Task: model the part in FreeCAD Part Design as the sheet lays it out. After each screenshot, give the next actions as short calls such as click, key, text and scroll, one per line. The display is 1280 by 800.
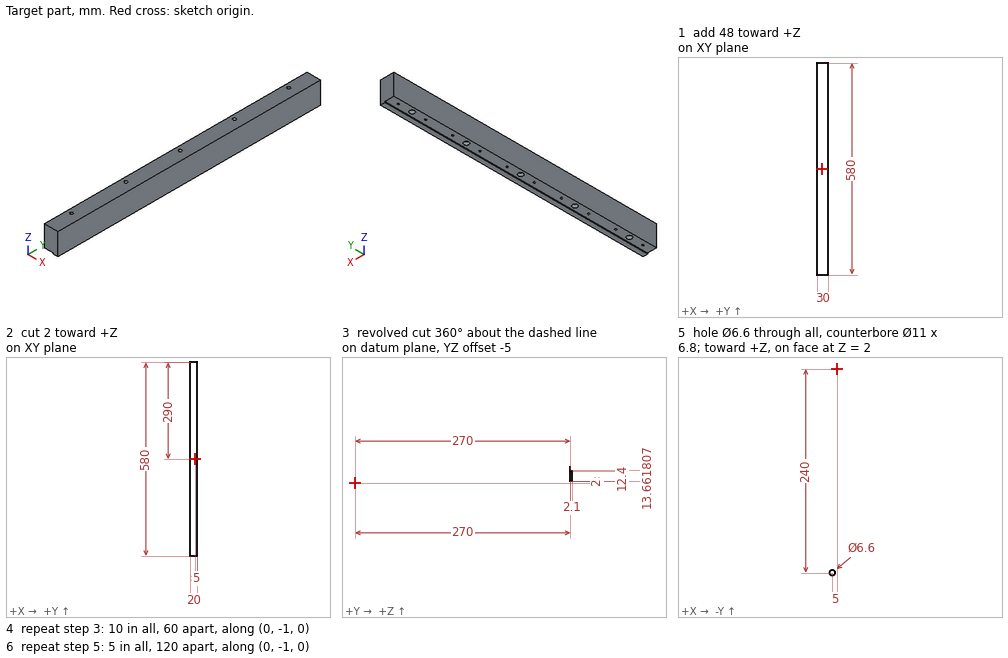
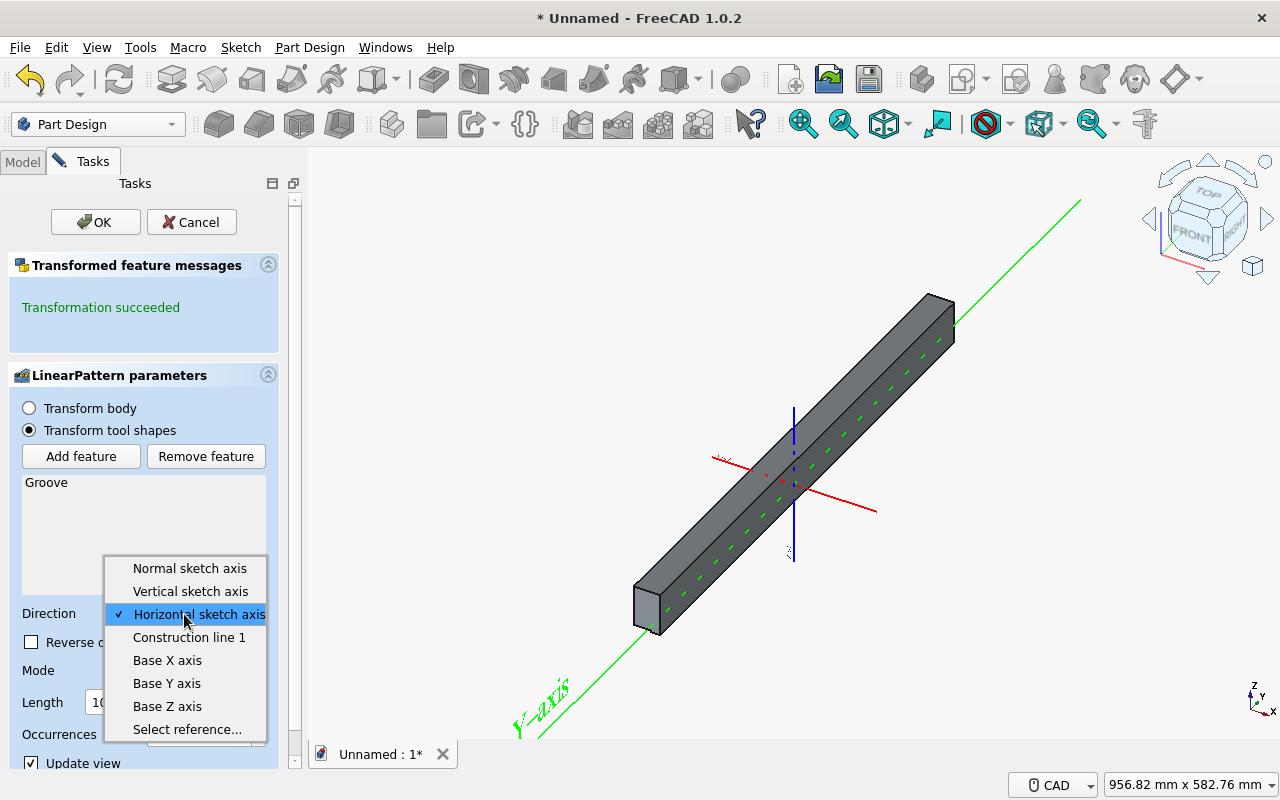
click(184, 684)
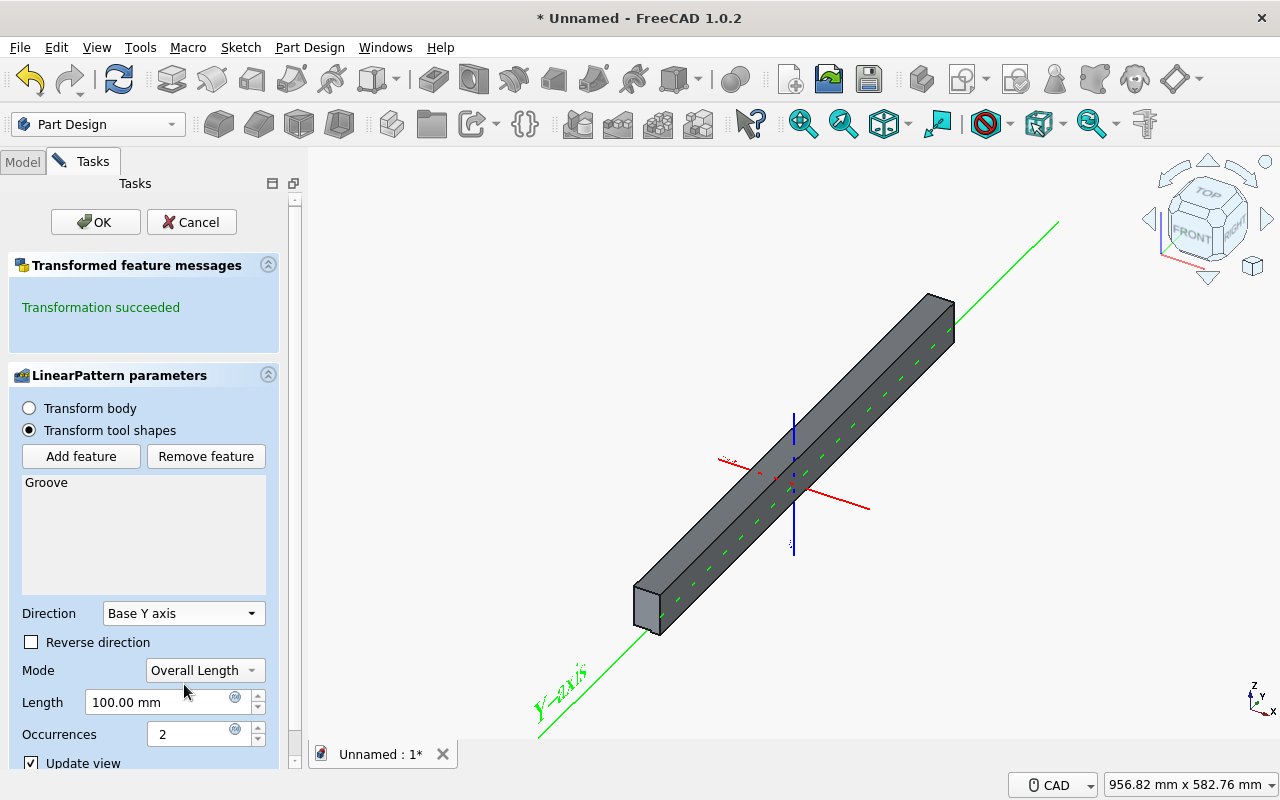
click(206, 670)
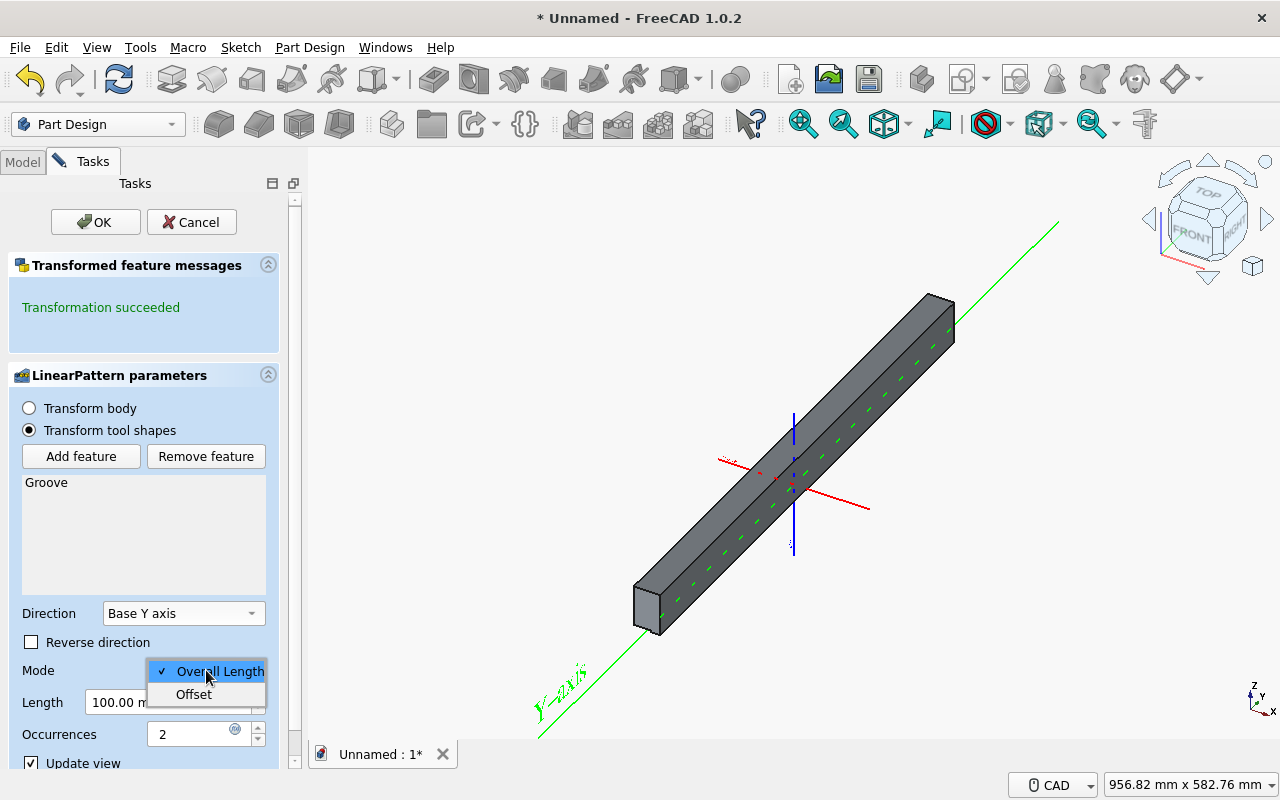
click(206, 694)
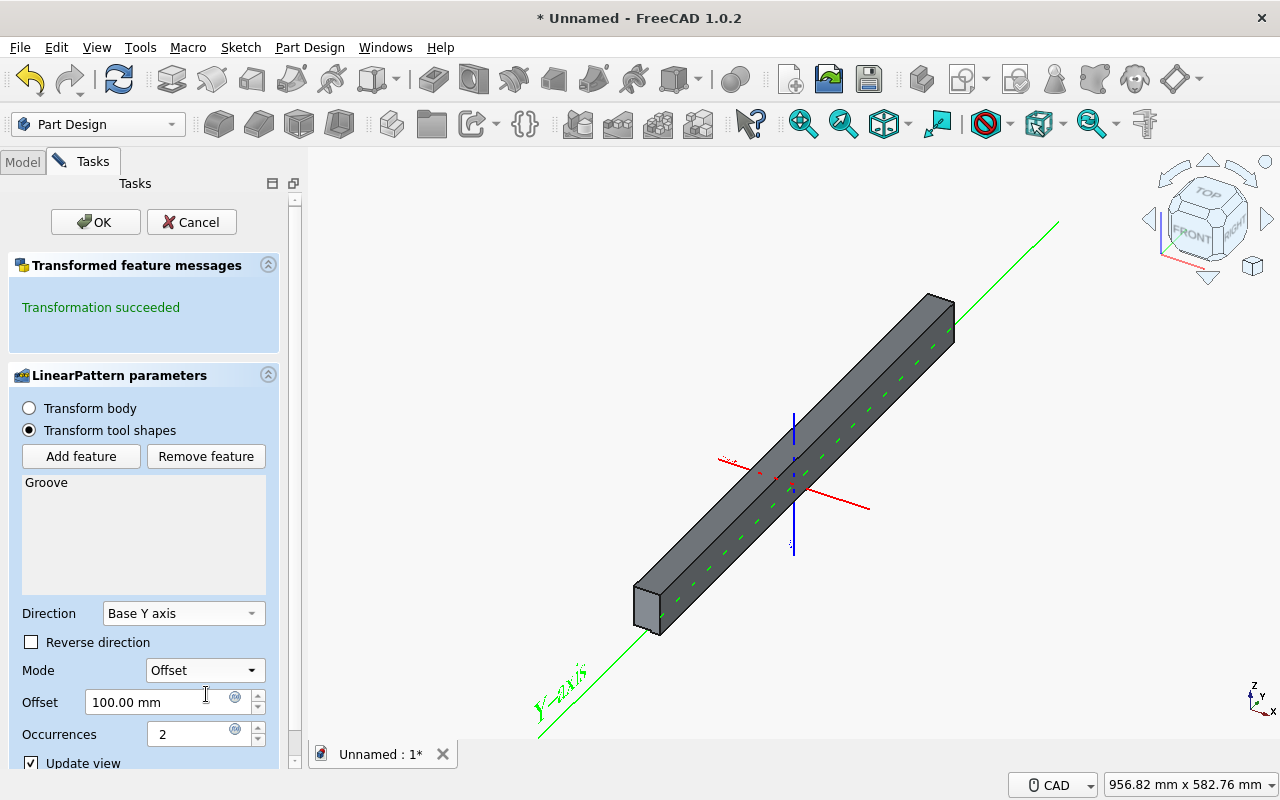
triple_click(168, 702)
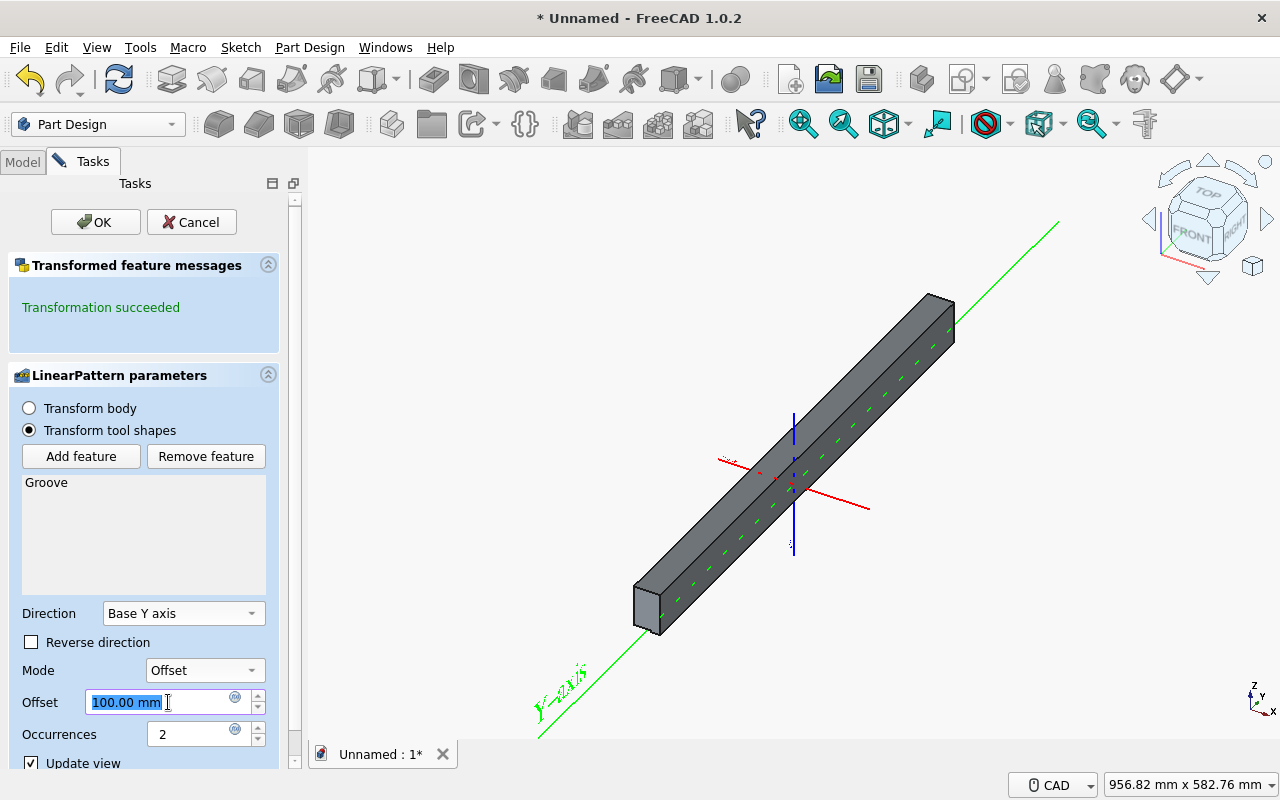
text(60)
key(Tab)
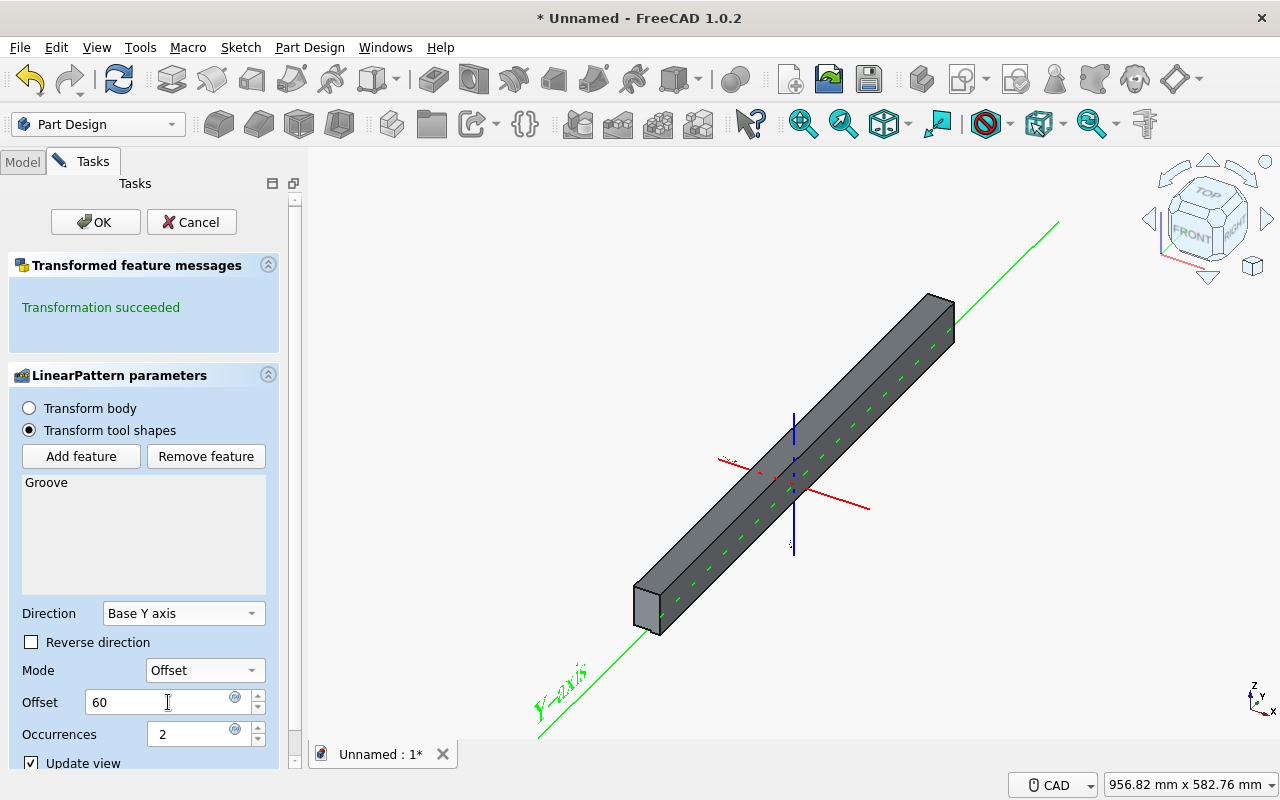
triple_click(198, 734)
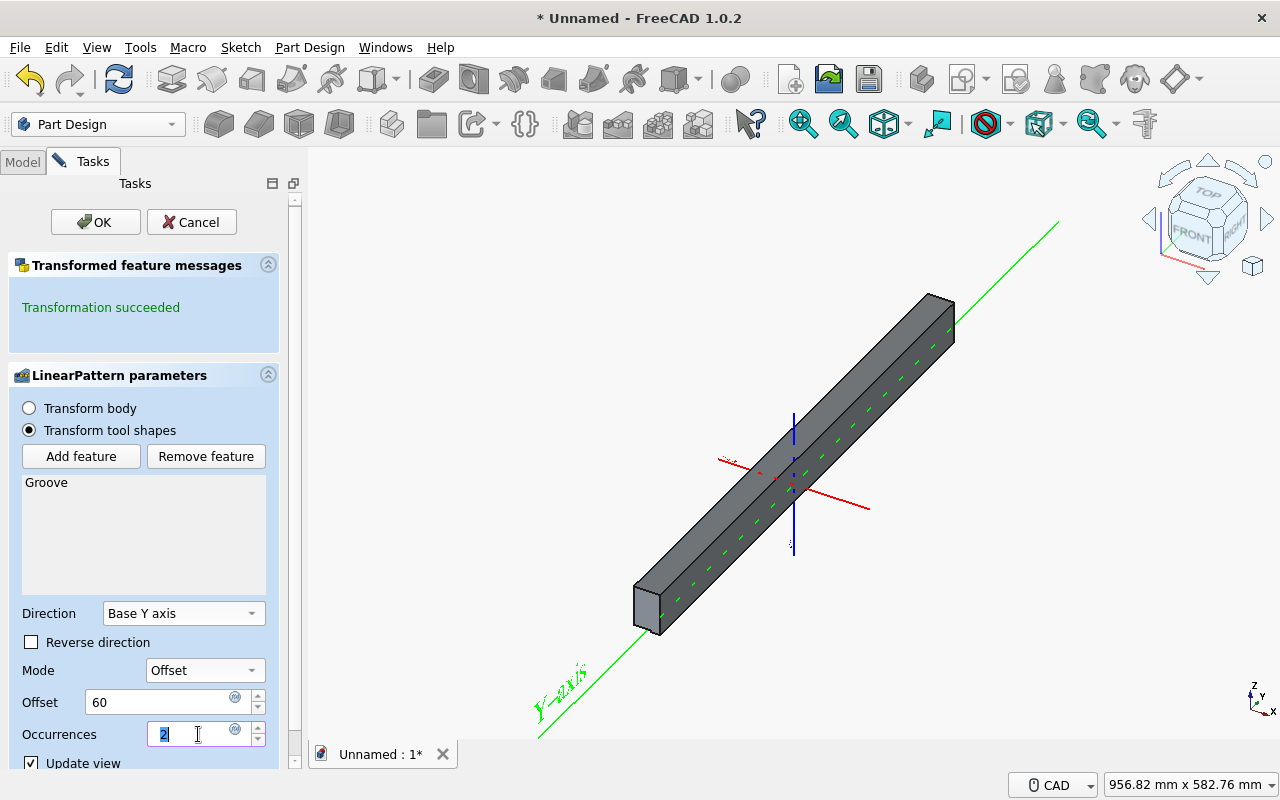
text(10)
key(Tab)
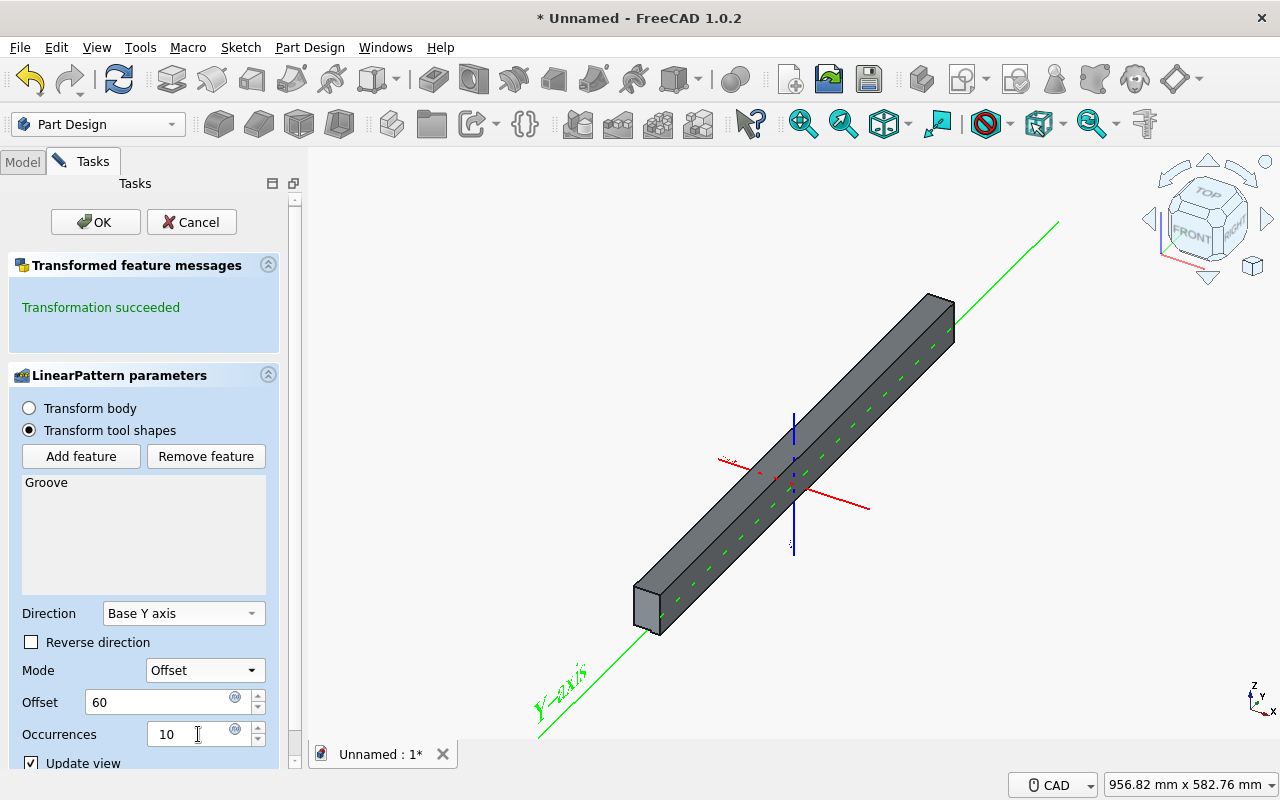
click(30, 642)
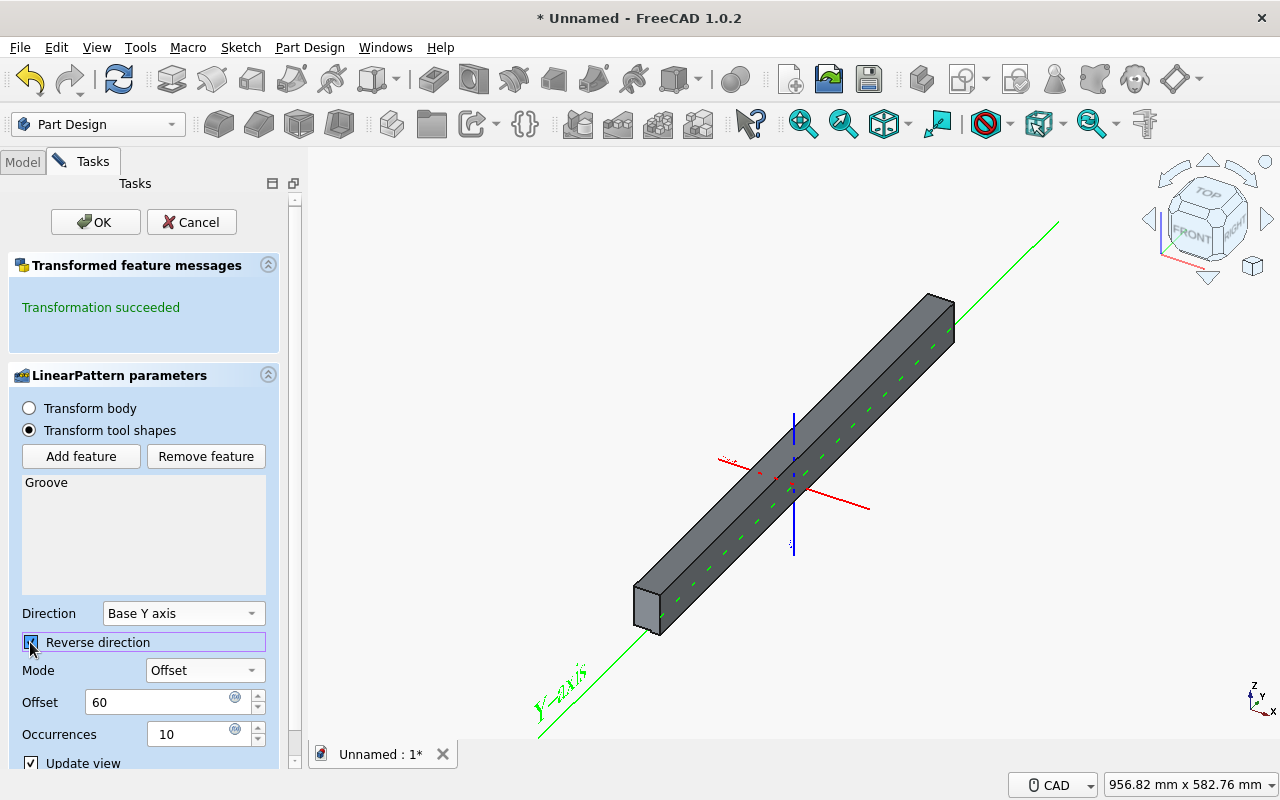
click(96, 222)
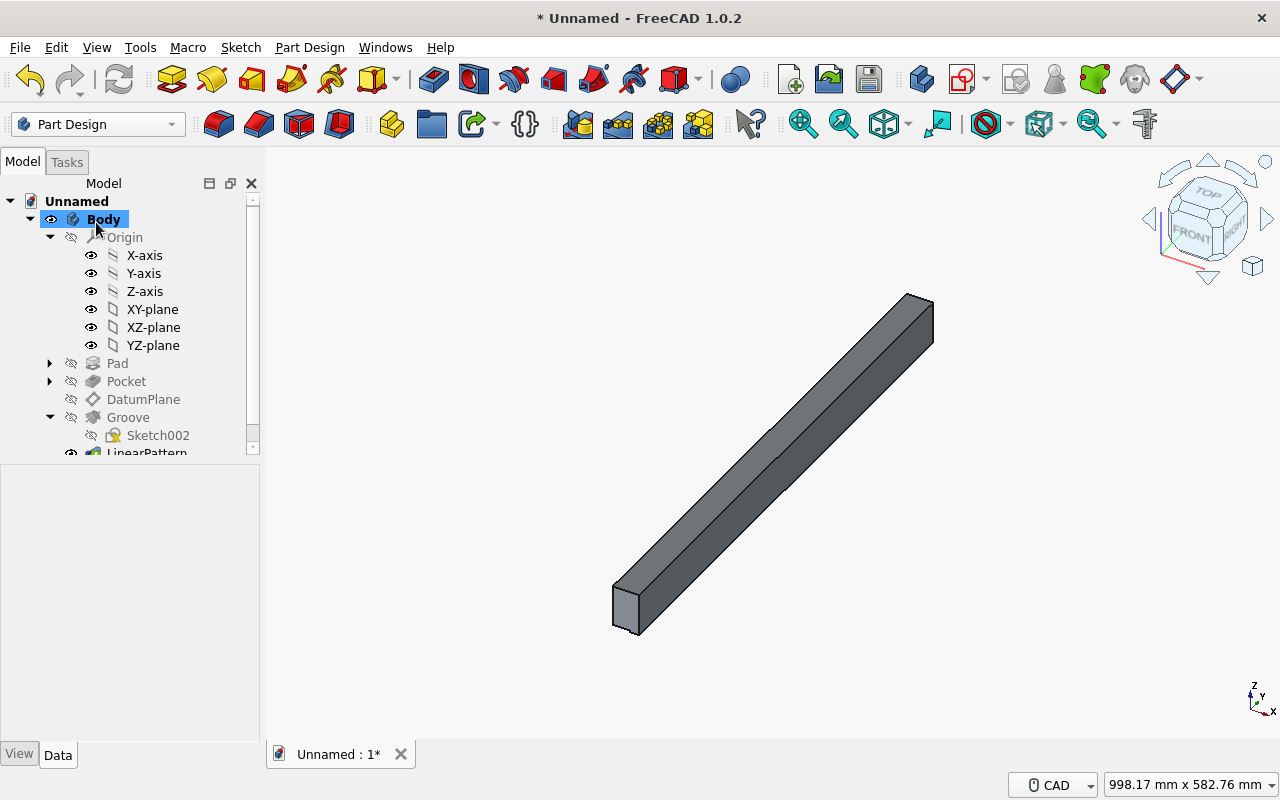
key(5)